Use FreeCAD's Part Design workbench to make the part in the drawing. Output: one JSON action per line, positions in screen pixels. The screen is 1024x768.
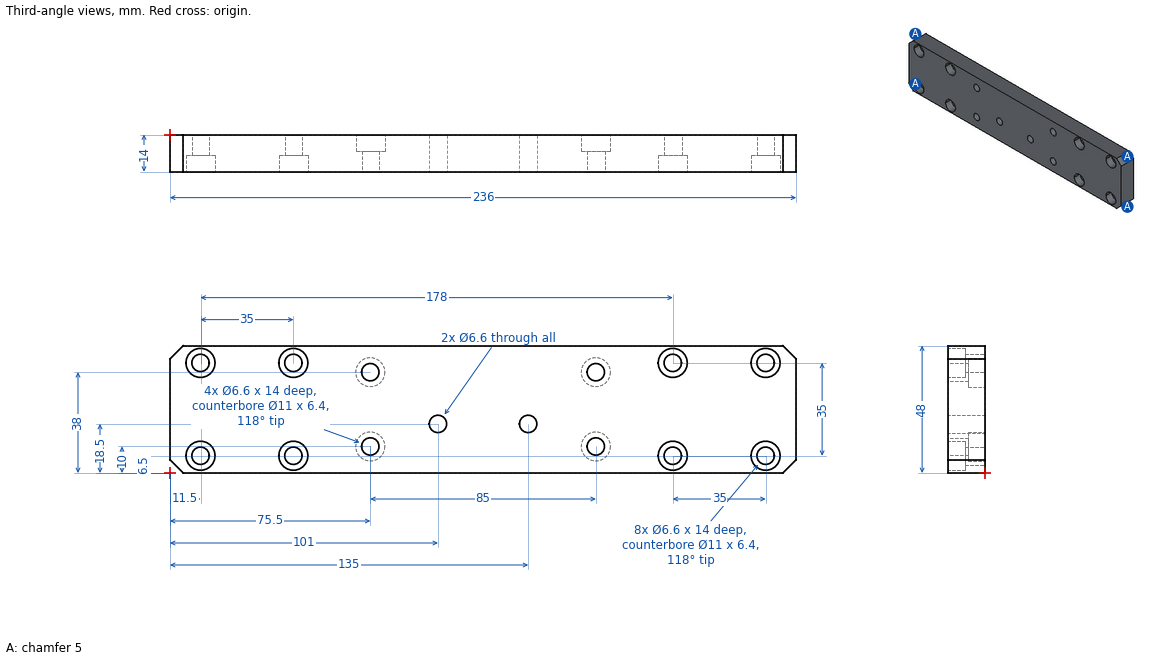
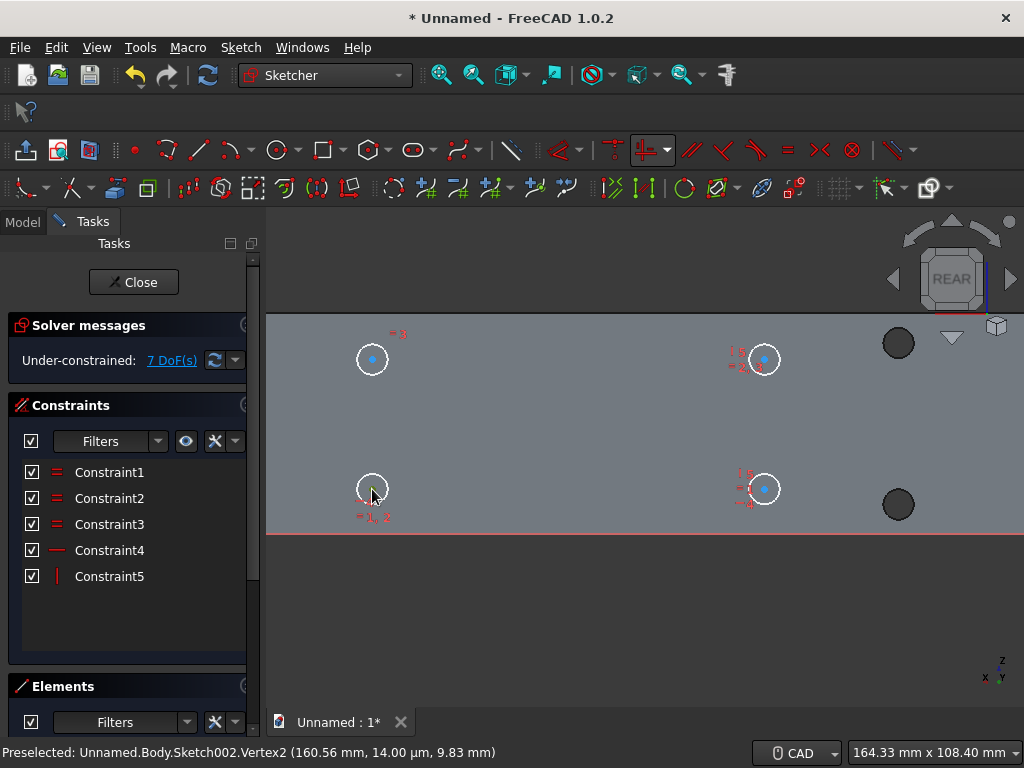
{"action": "left_click", "coordinate": [372, 360]}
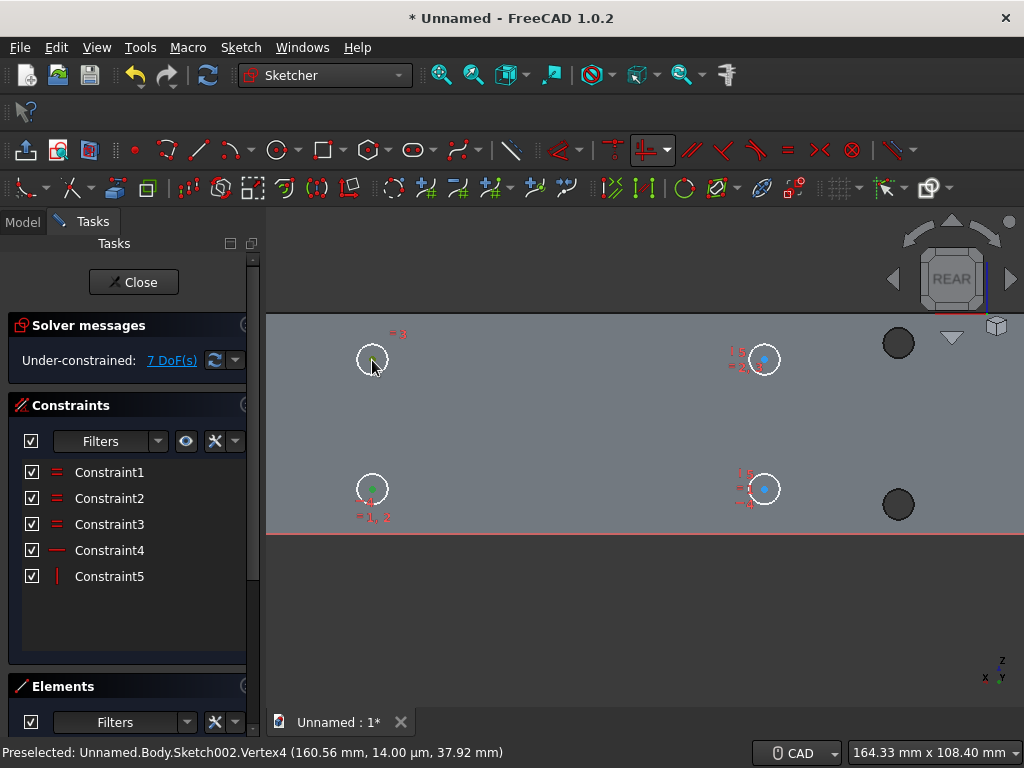
{"action": "left_click", "coordinate": [670, 150]}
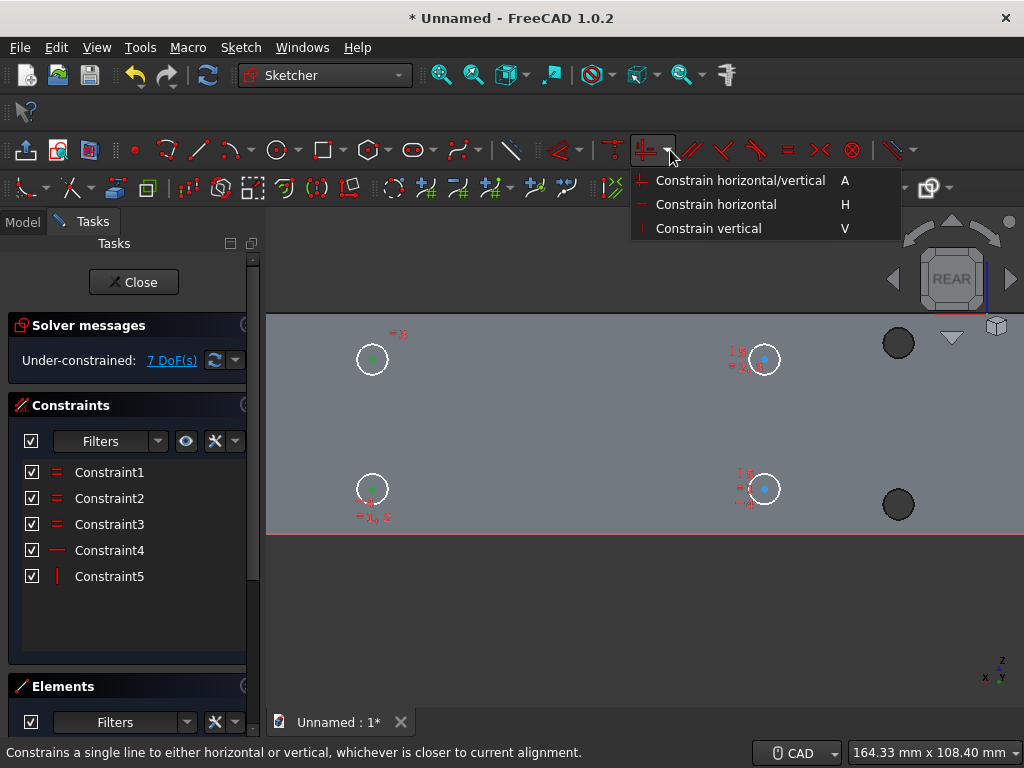
{"action": "left_click", "coordinate": [766, 228]}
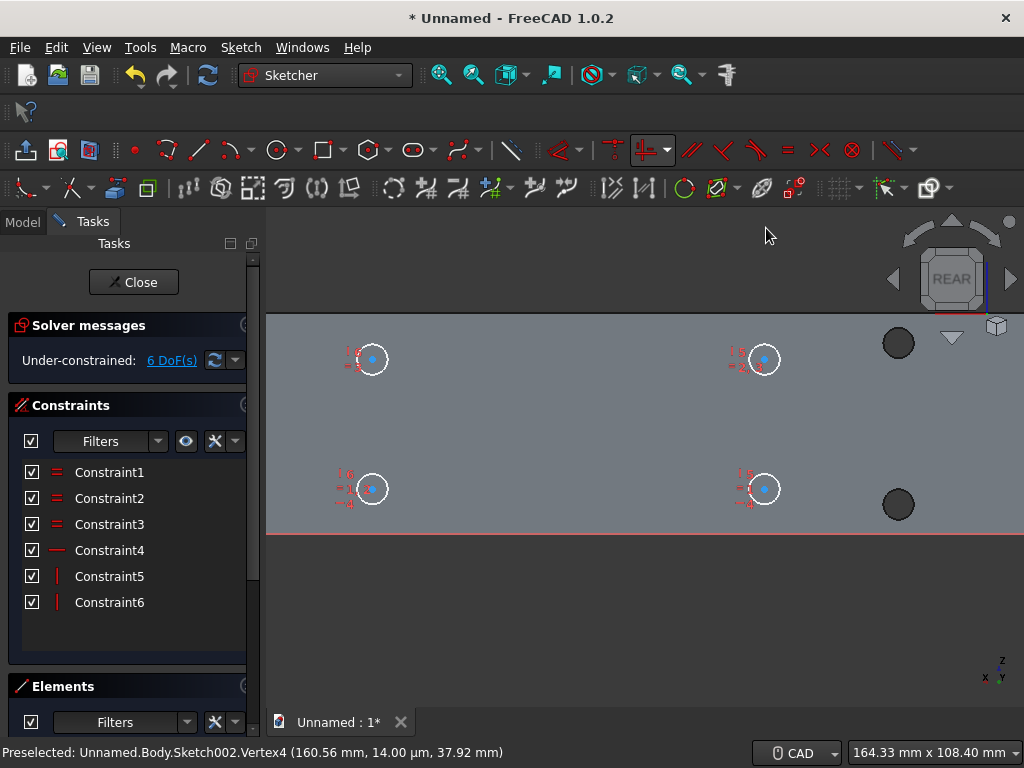
{"action": "left_click", "coordinate": [765, 360]}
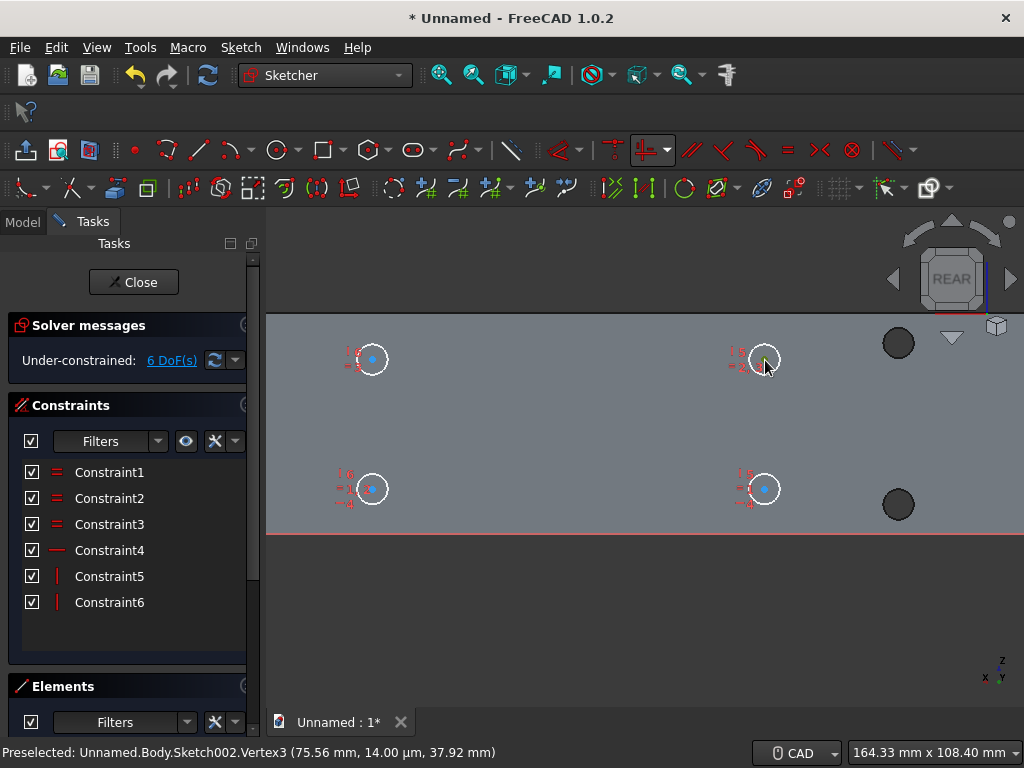
{"action": "left_click", "coordinate": [372, 360]}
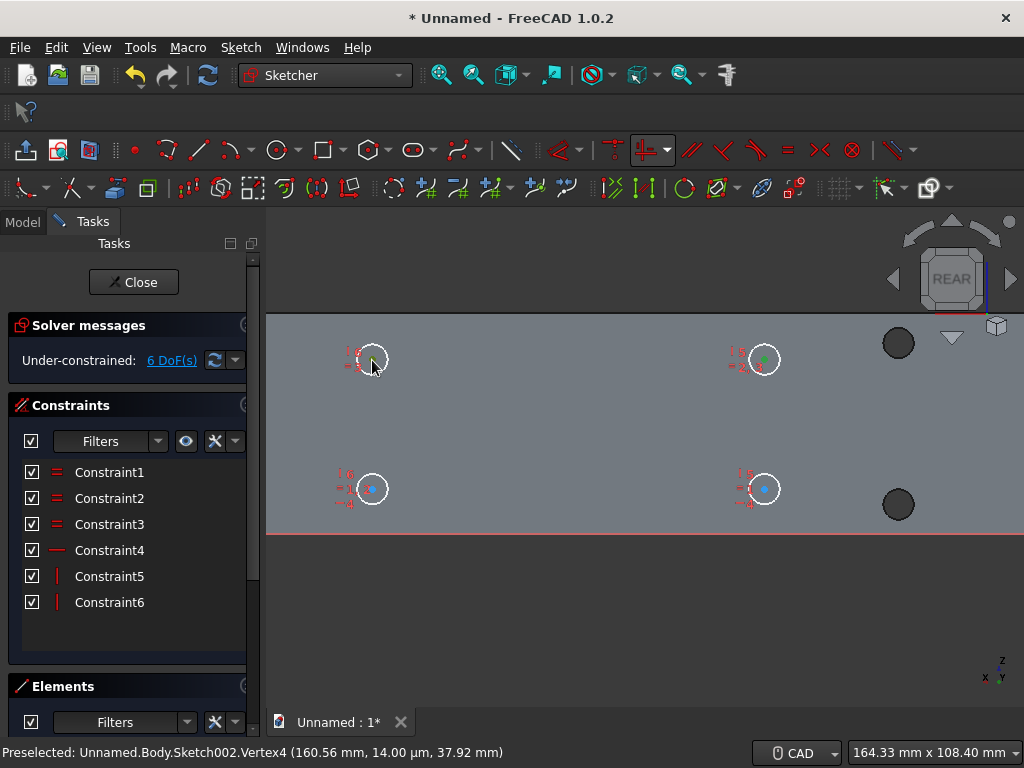
{"action": "left_click", "coordinate": [670, 150]}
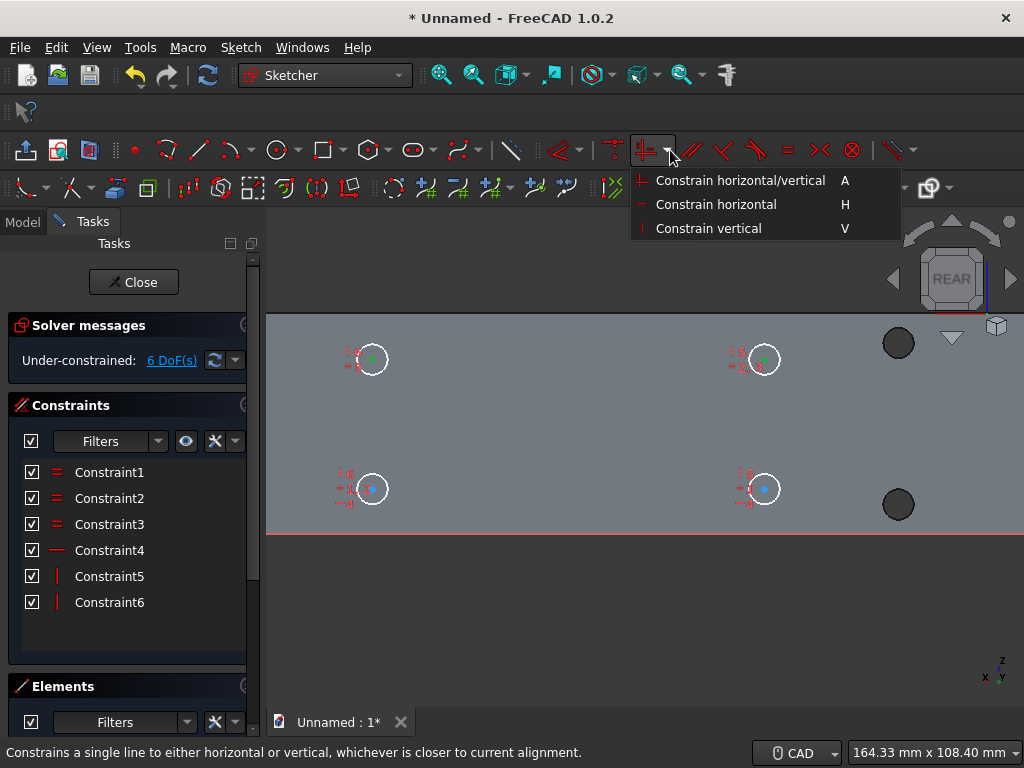
{"action": "left_click", "coordinate": [766, 204]}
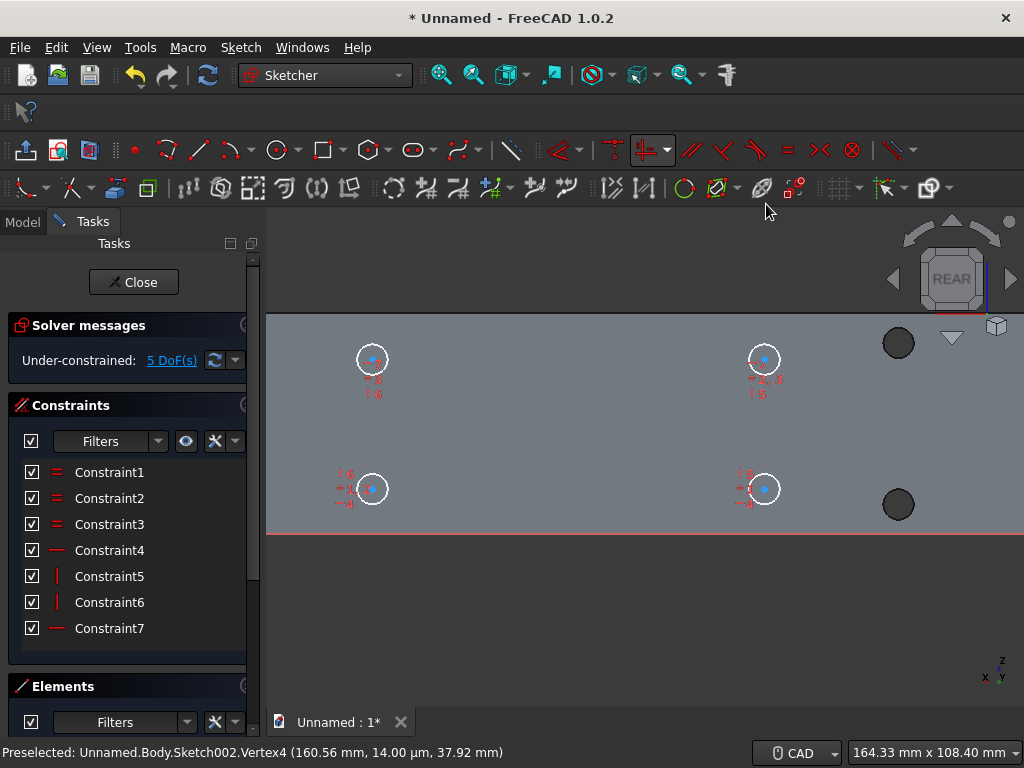
{"action": "left_click", "coordinate": [558, 150]}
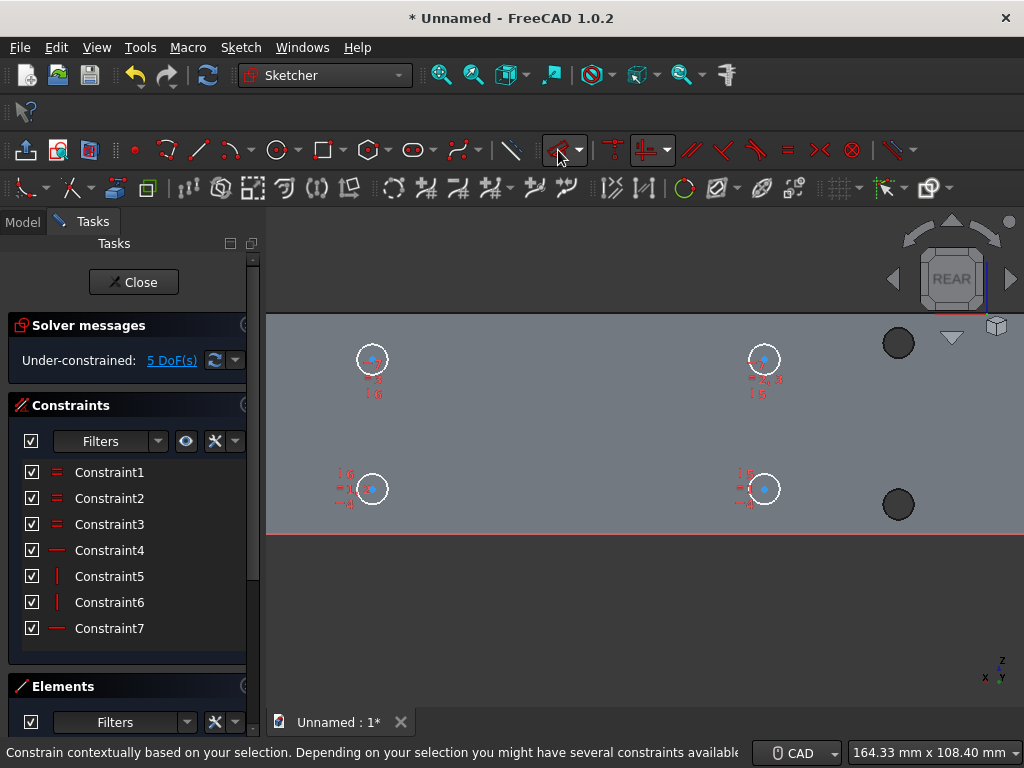
{"action": "scroll", "coordinate": [775, 478], "scroll_direction": "up", "scroll_amount": 2}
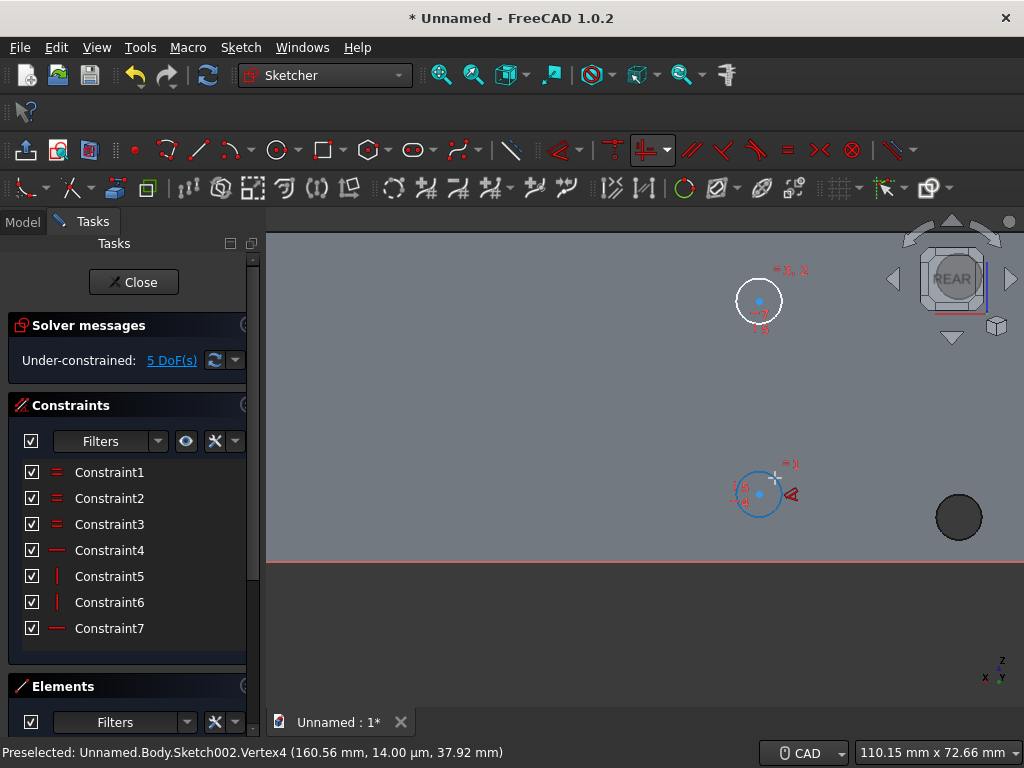
{"action": "left_click", "coordinate": [775, 478]}
{"action": "left_click", "coordinate": [797, 455]}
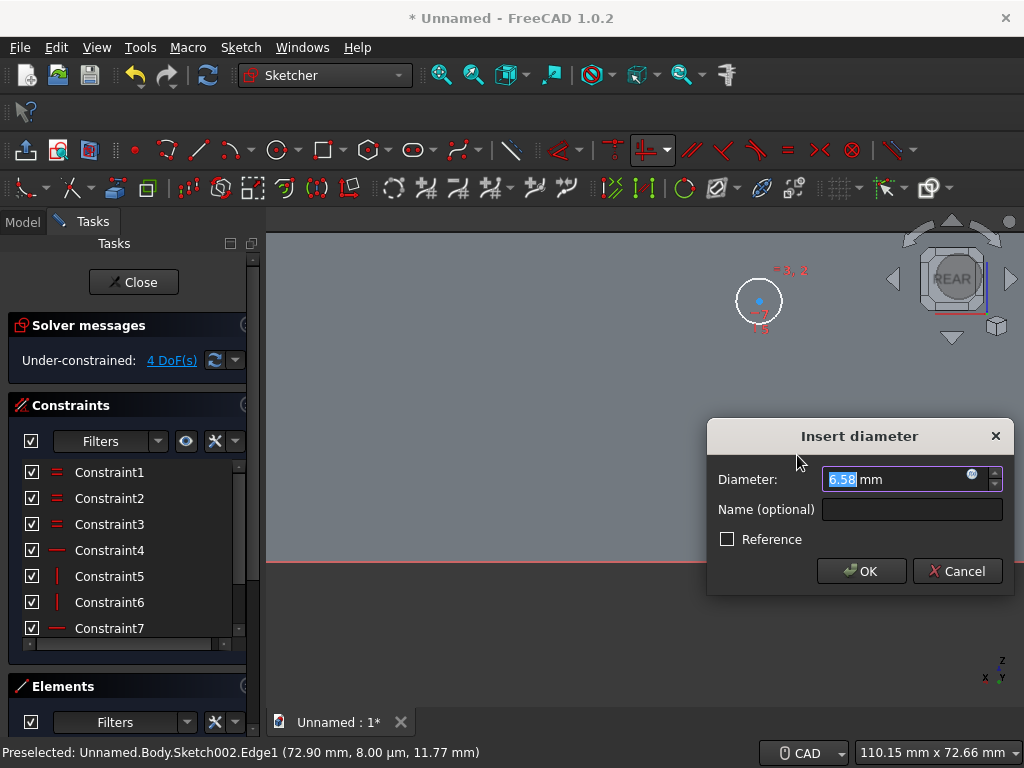
{"action": "type", "text": "6.6"}
{"action": "key", "text": "Return"}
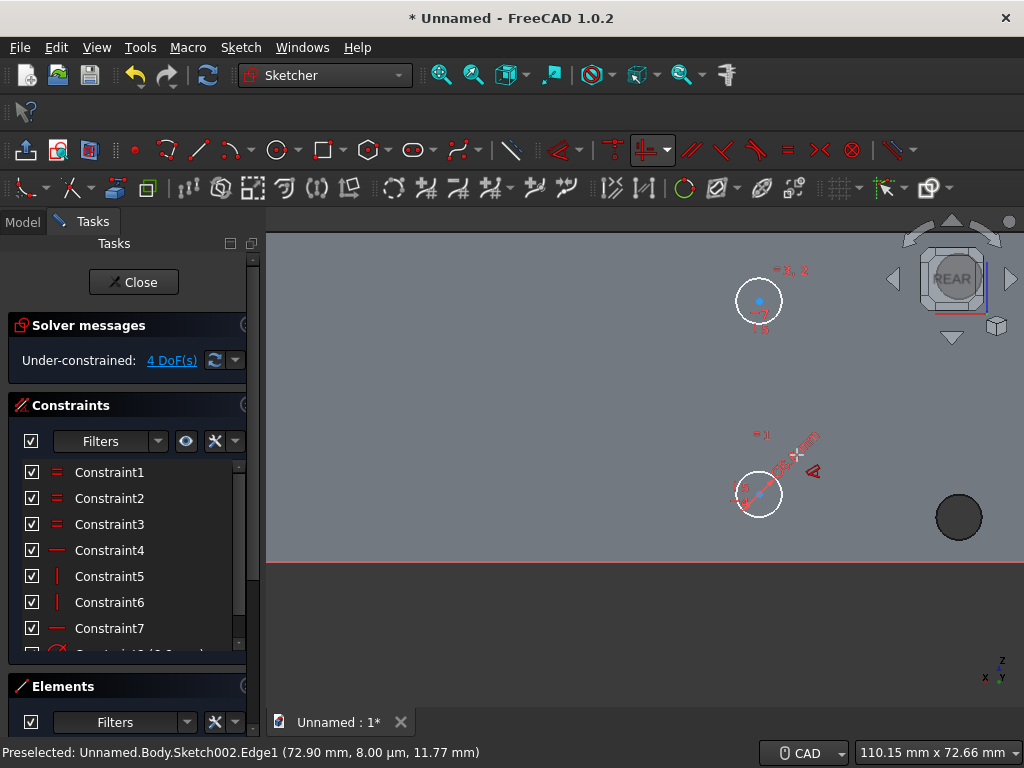
{"action": "left_click", "coordinate": [759, 494]}
{"action": "left_click", "coordinate": [725, 528]}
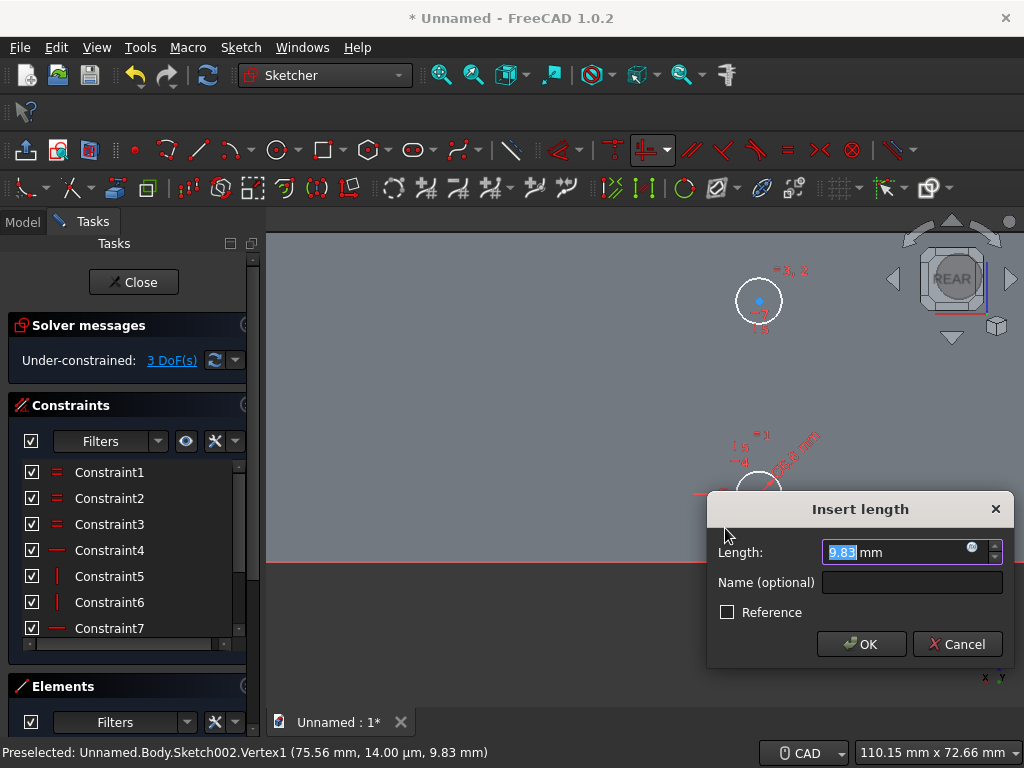
{"action": "type", "text": "10"}
{"action": "key", "text": "Return"}